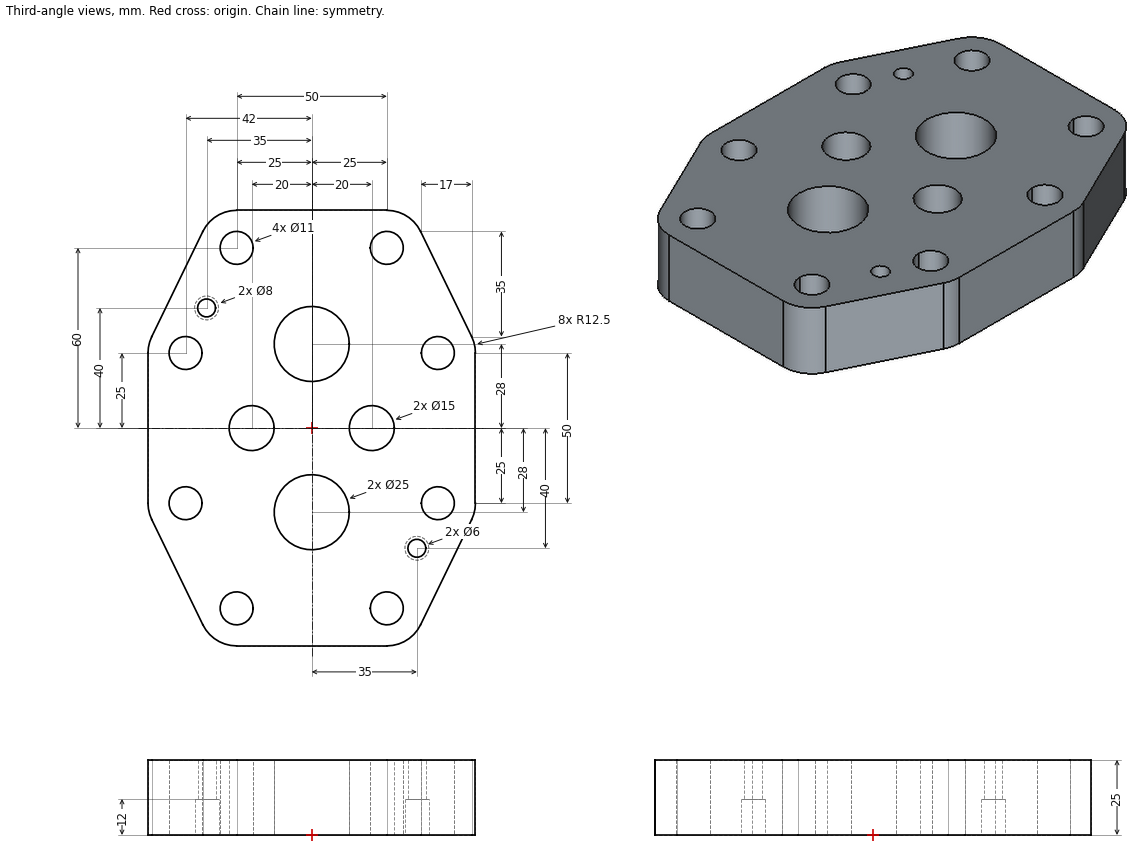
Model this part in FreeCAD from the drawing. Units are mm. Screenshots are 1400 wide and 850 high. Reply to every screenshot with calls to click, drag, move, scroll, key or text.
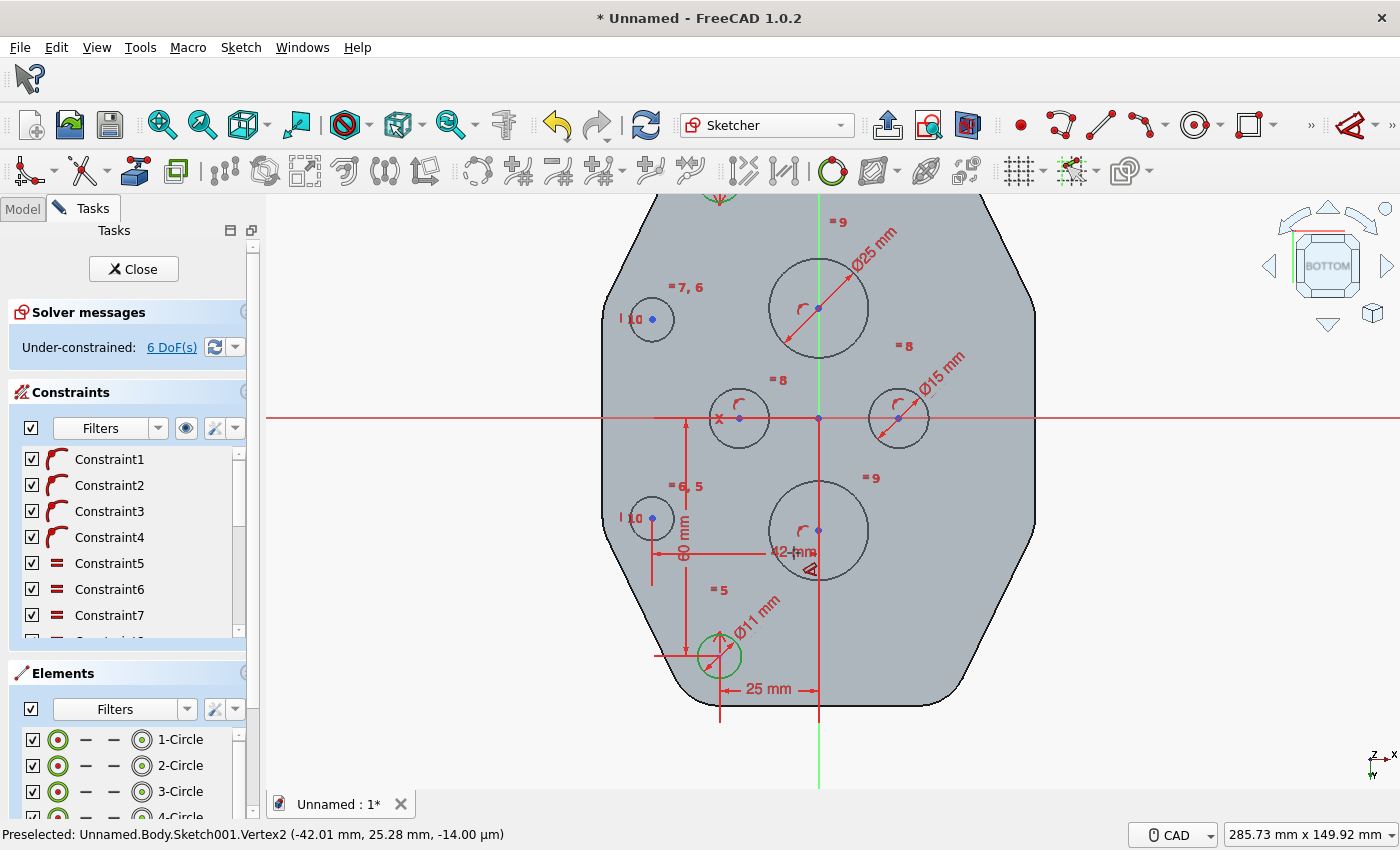
click(652, 519)
click(618, 469)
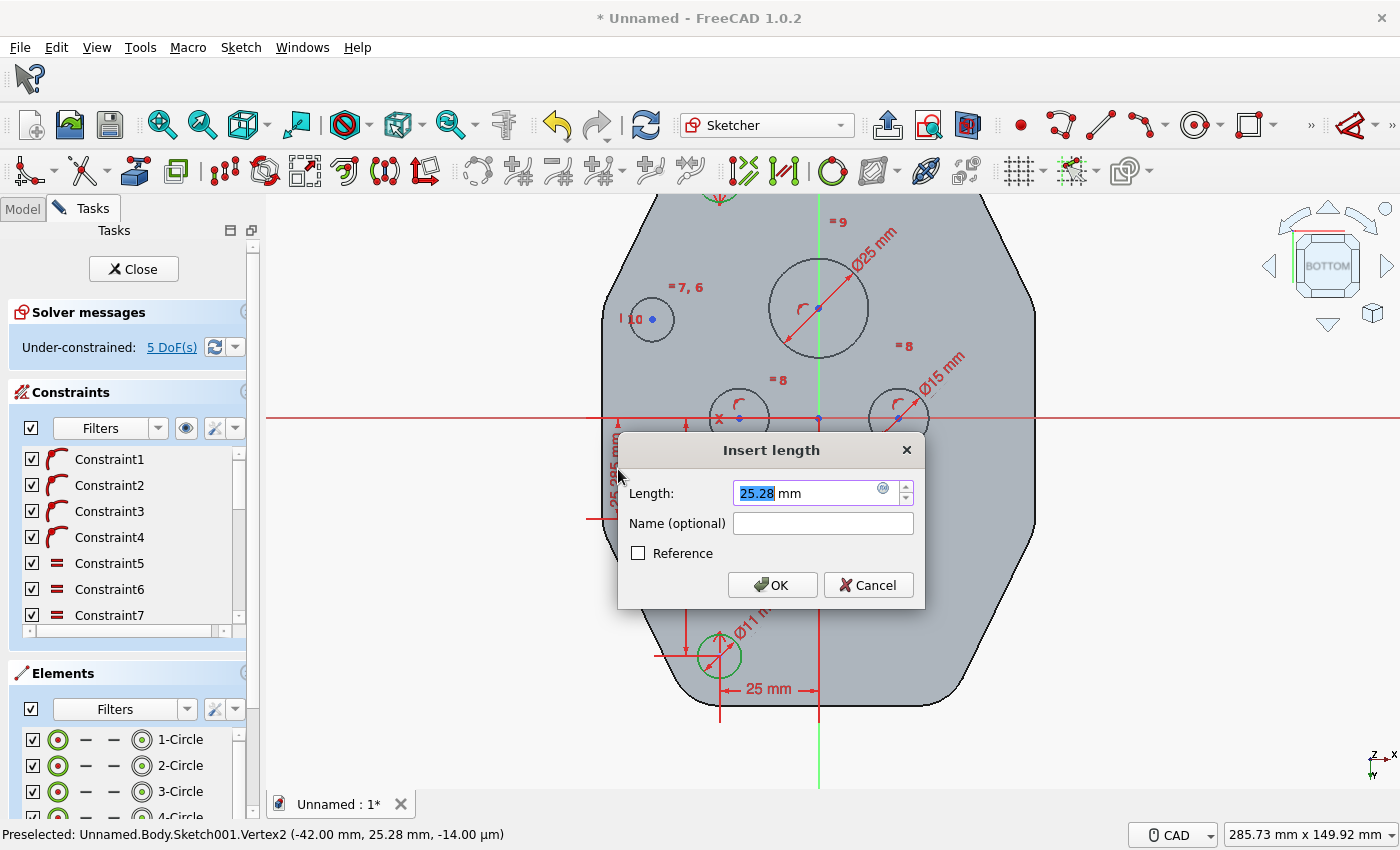
text(25)
key(Return)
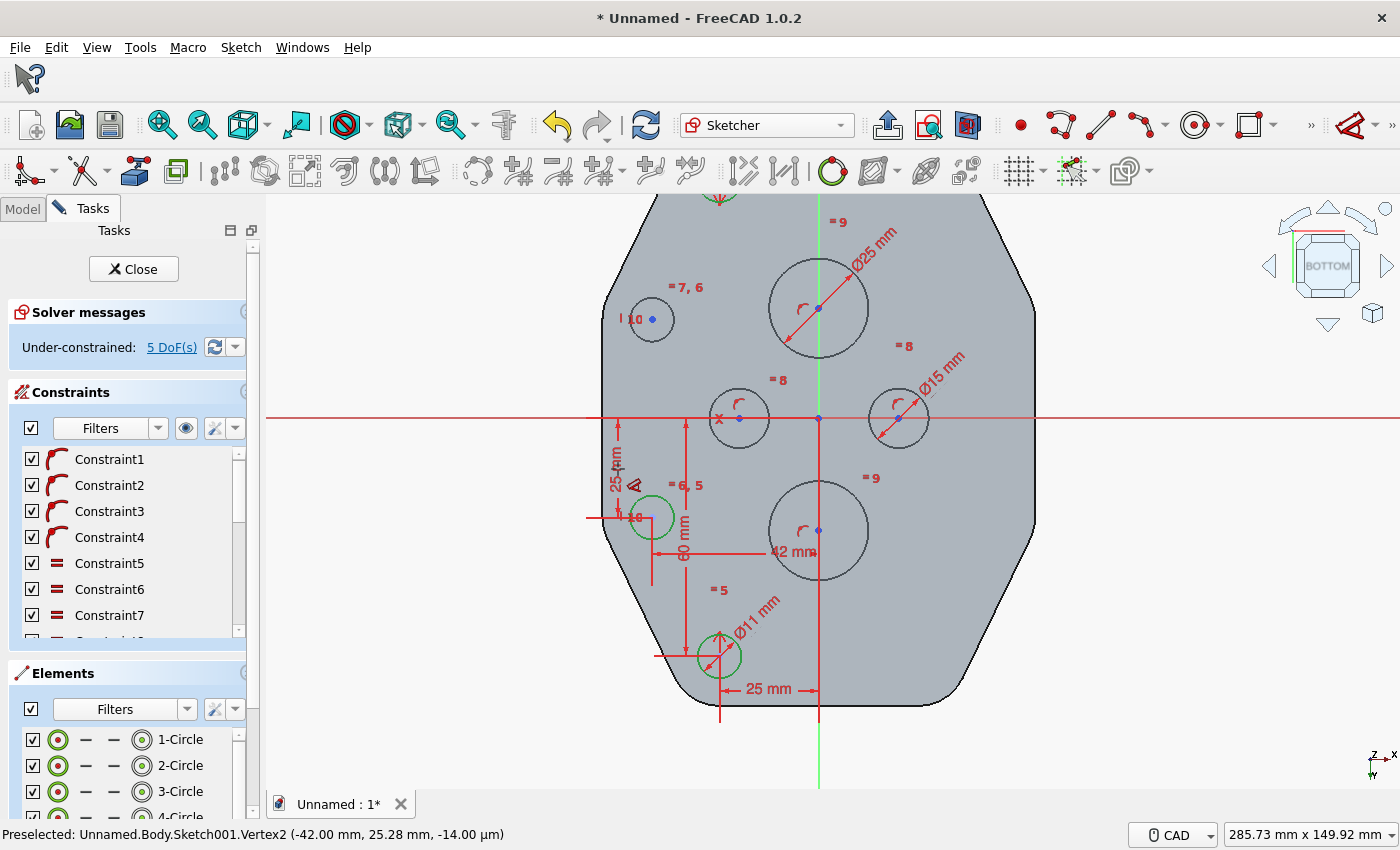
click(652, 320)
click(618, 369)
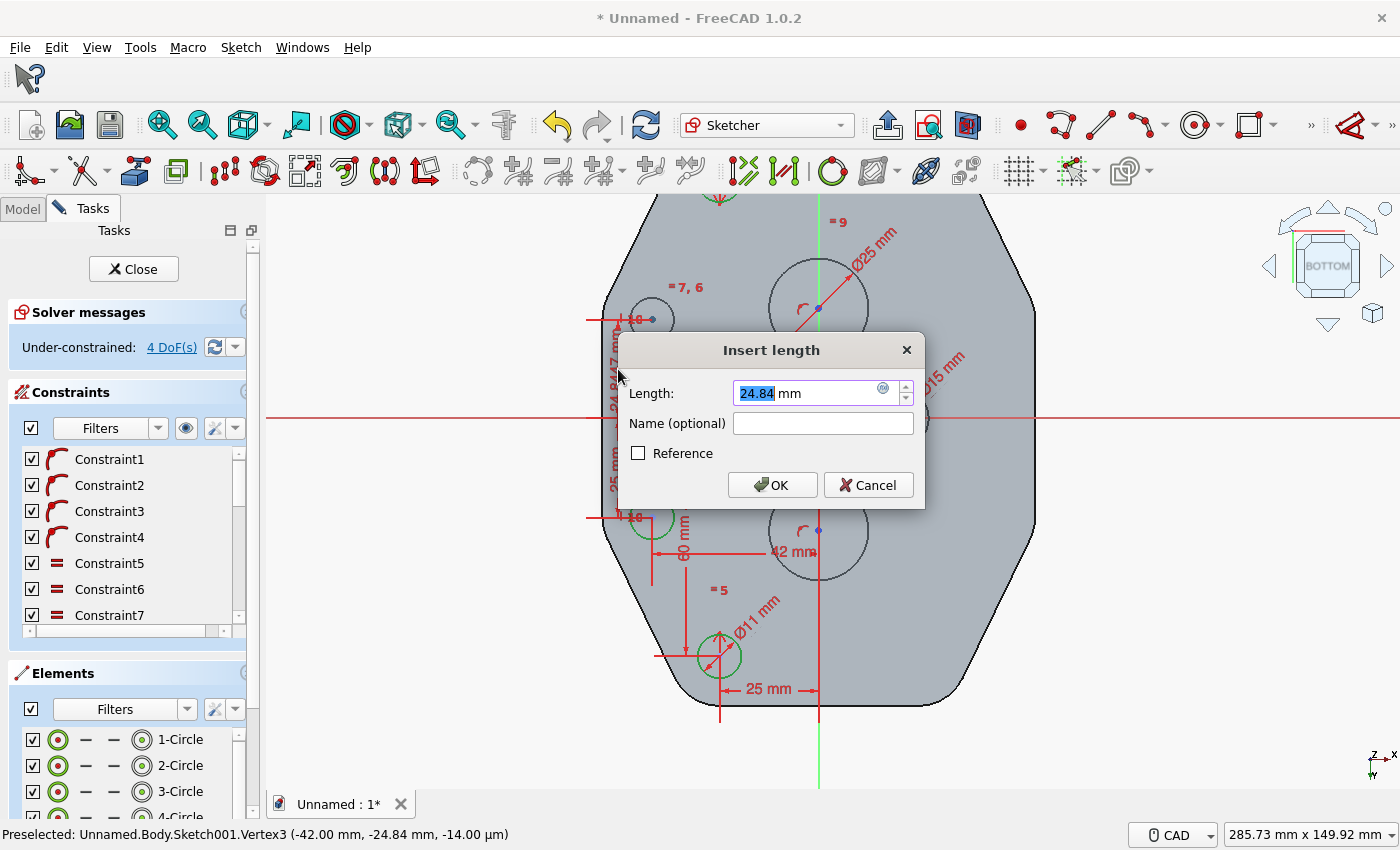
text(25)
key(Return)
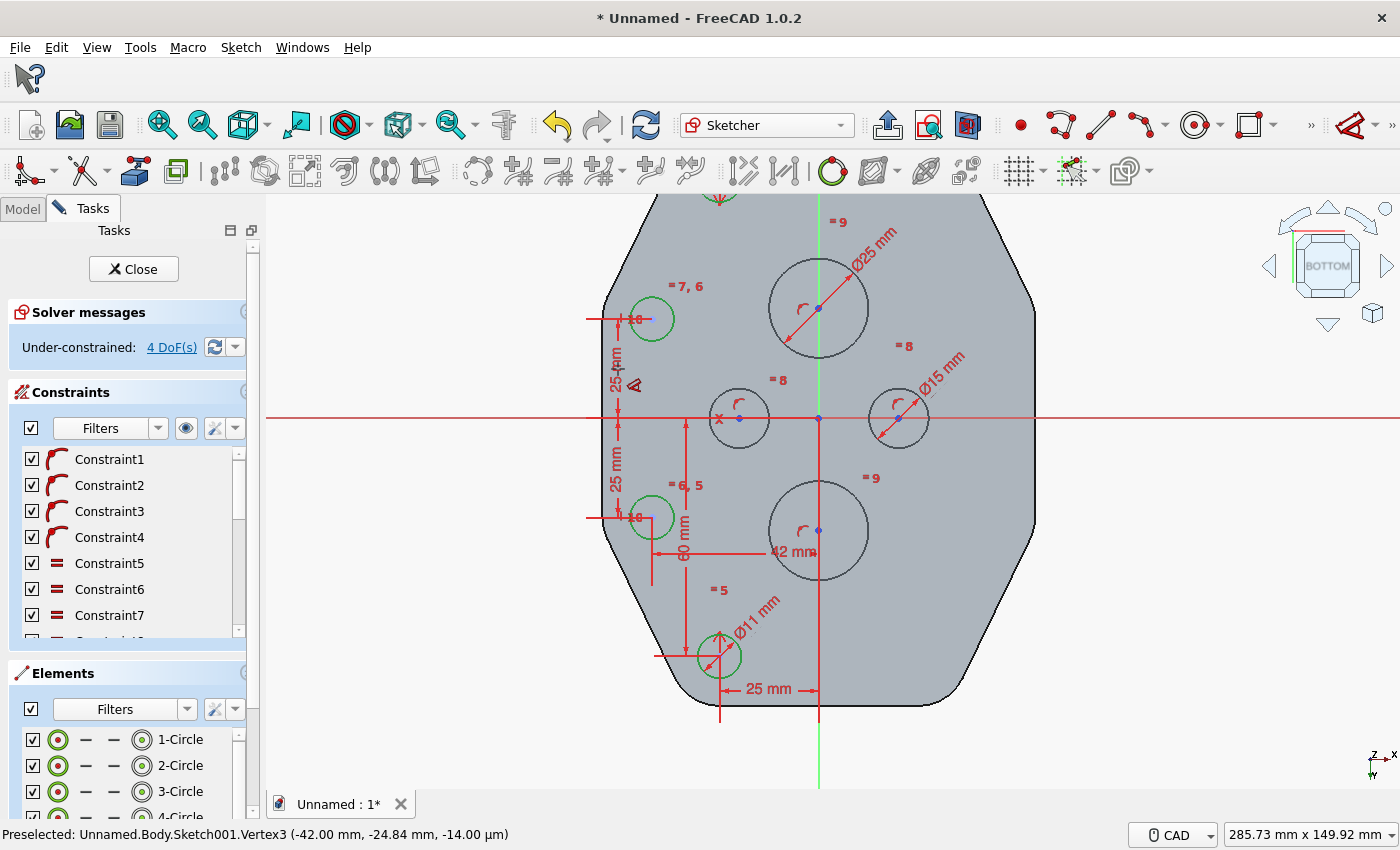
click(819, 308)
click(853, 363)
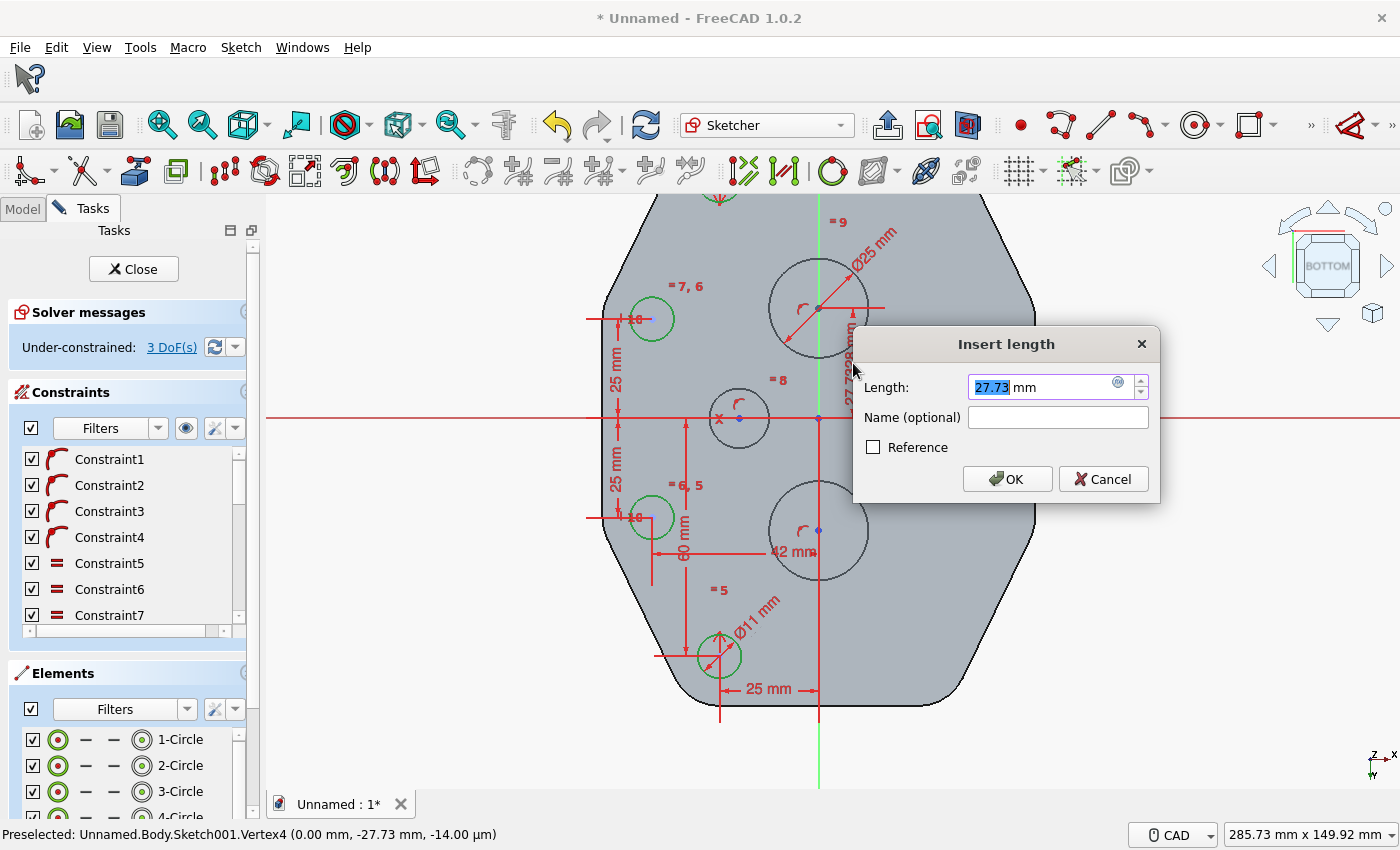
text(28)
key(Return)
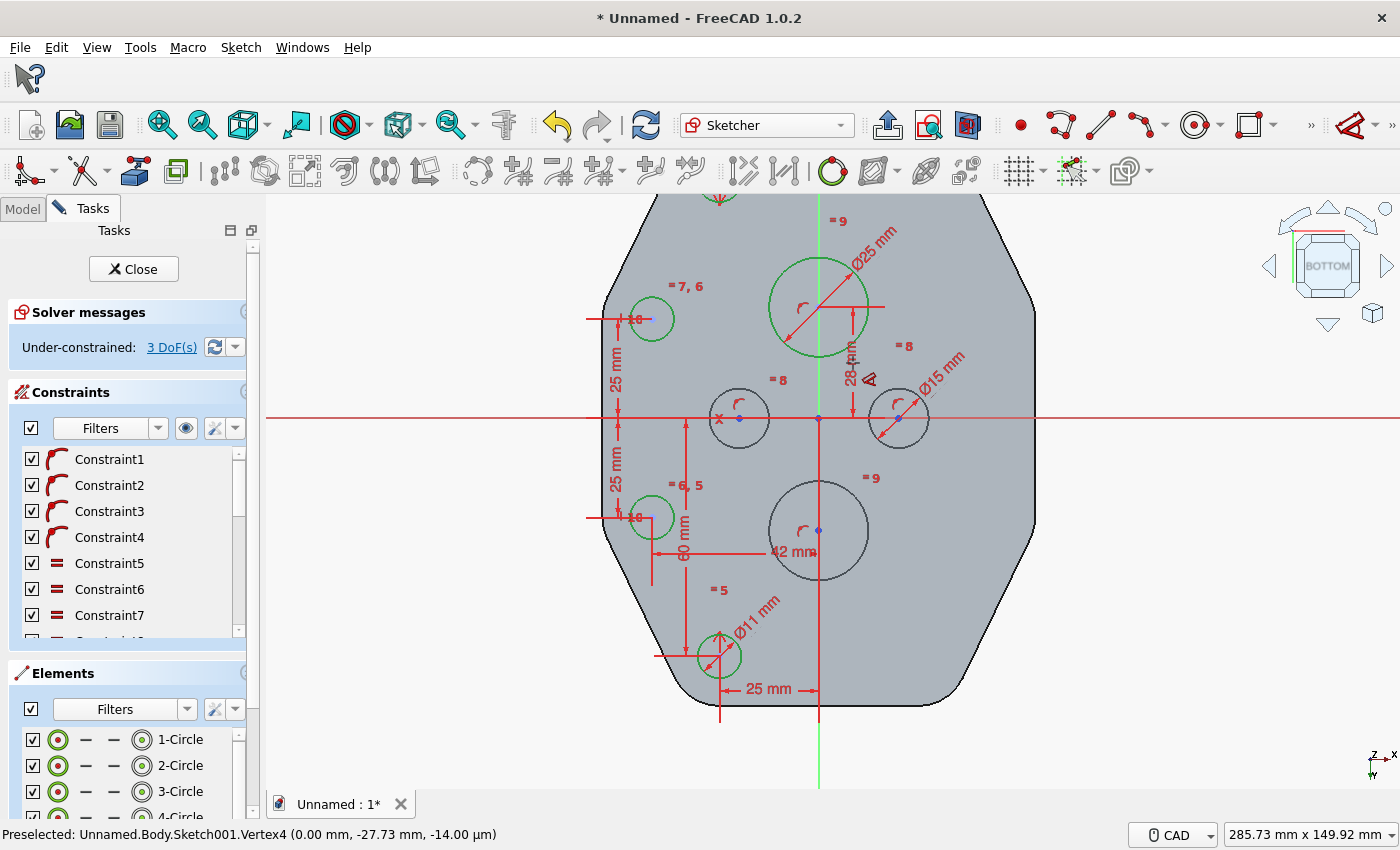
click(899, 418)
click(859, 452)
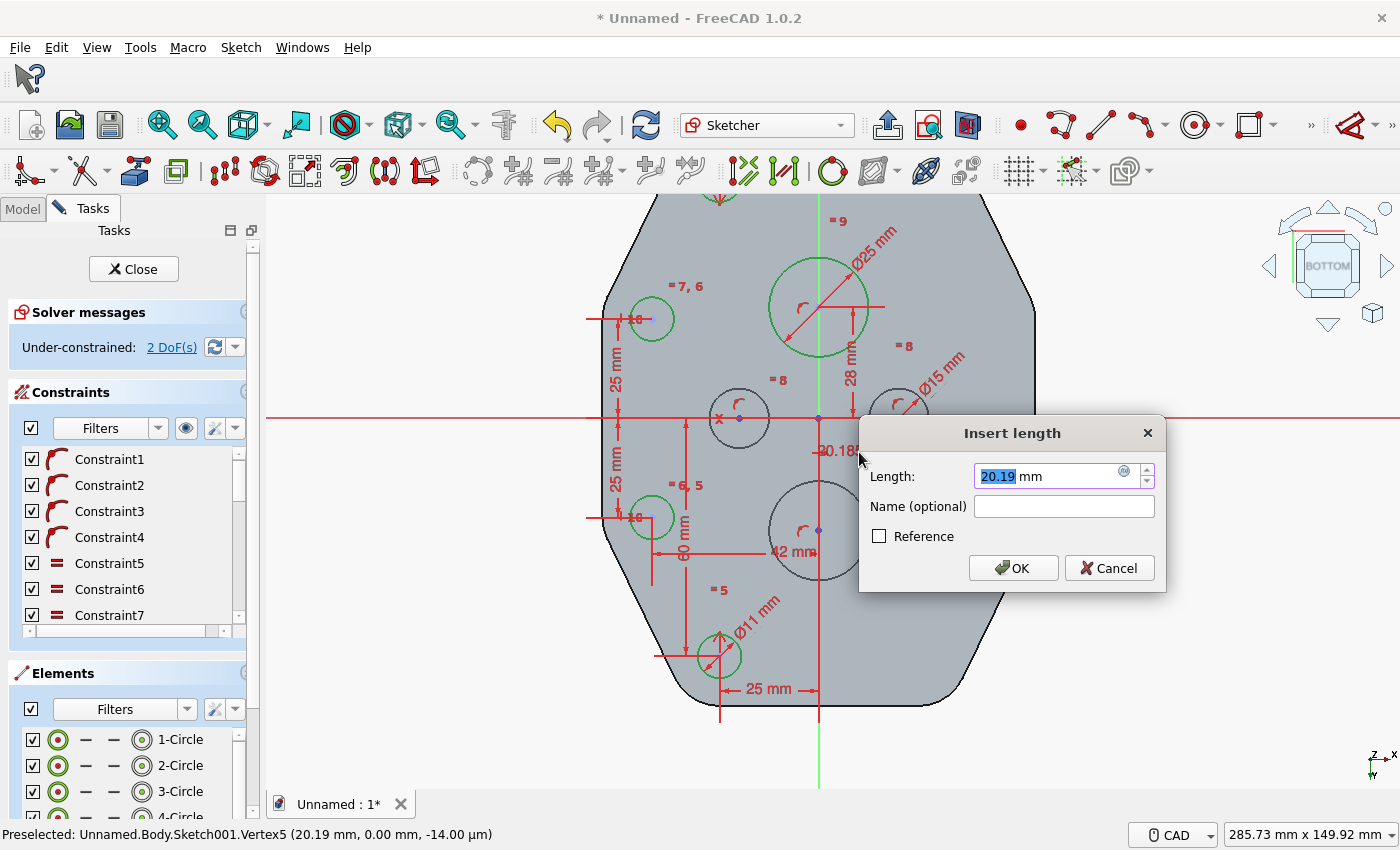
text(20)
key(Return)